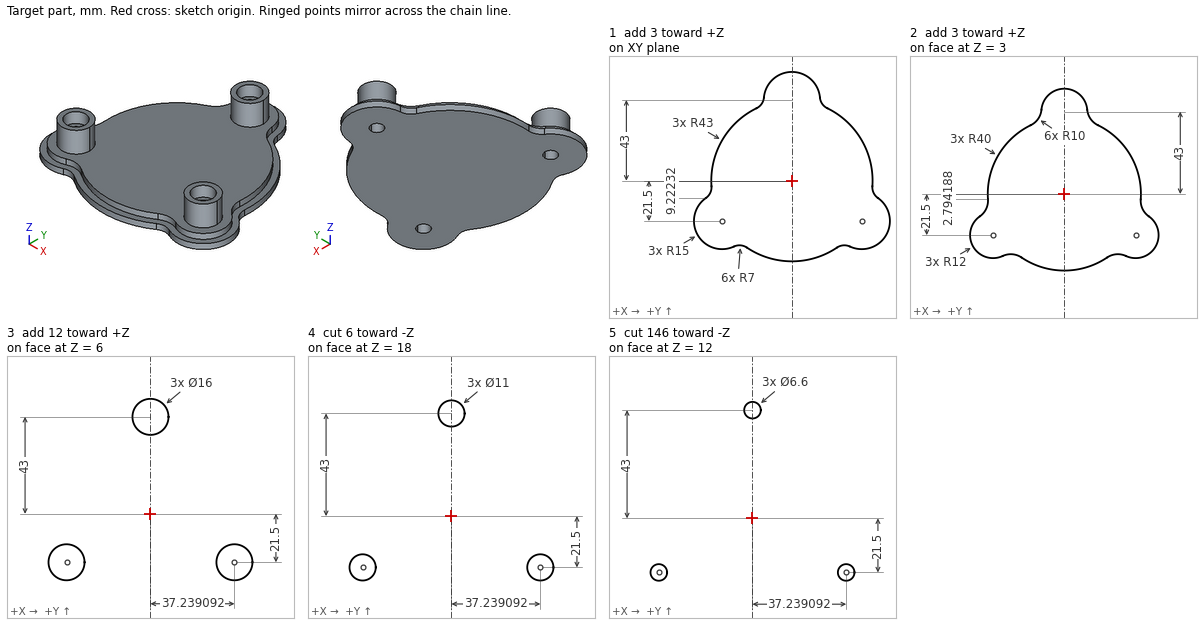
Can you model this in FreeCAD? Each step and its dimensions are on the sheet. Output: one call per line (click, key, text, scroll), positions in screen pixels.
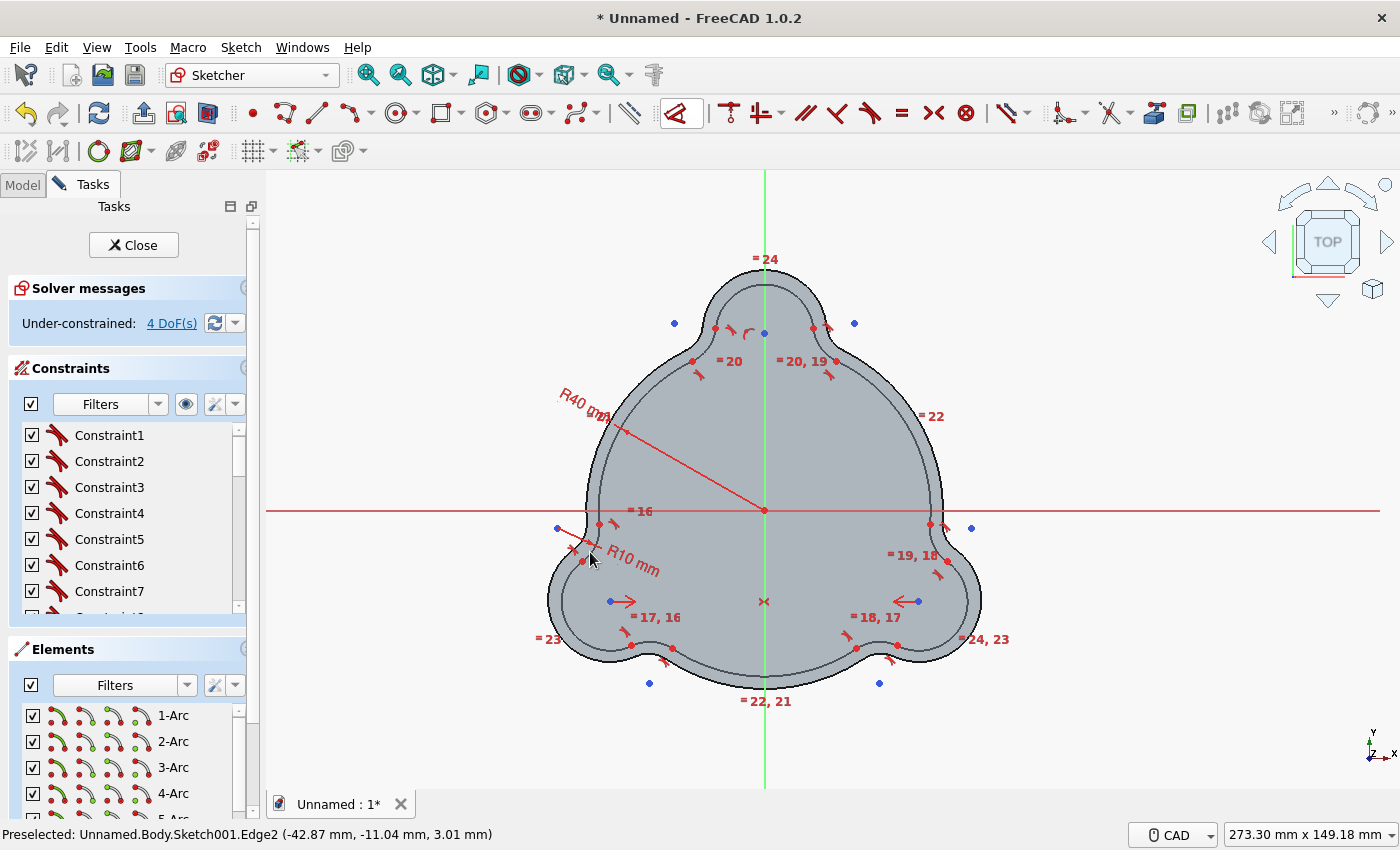
click(562, 599)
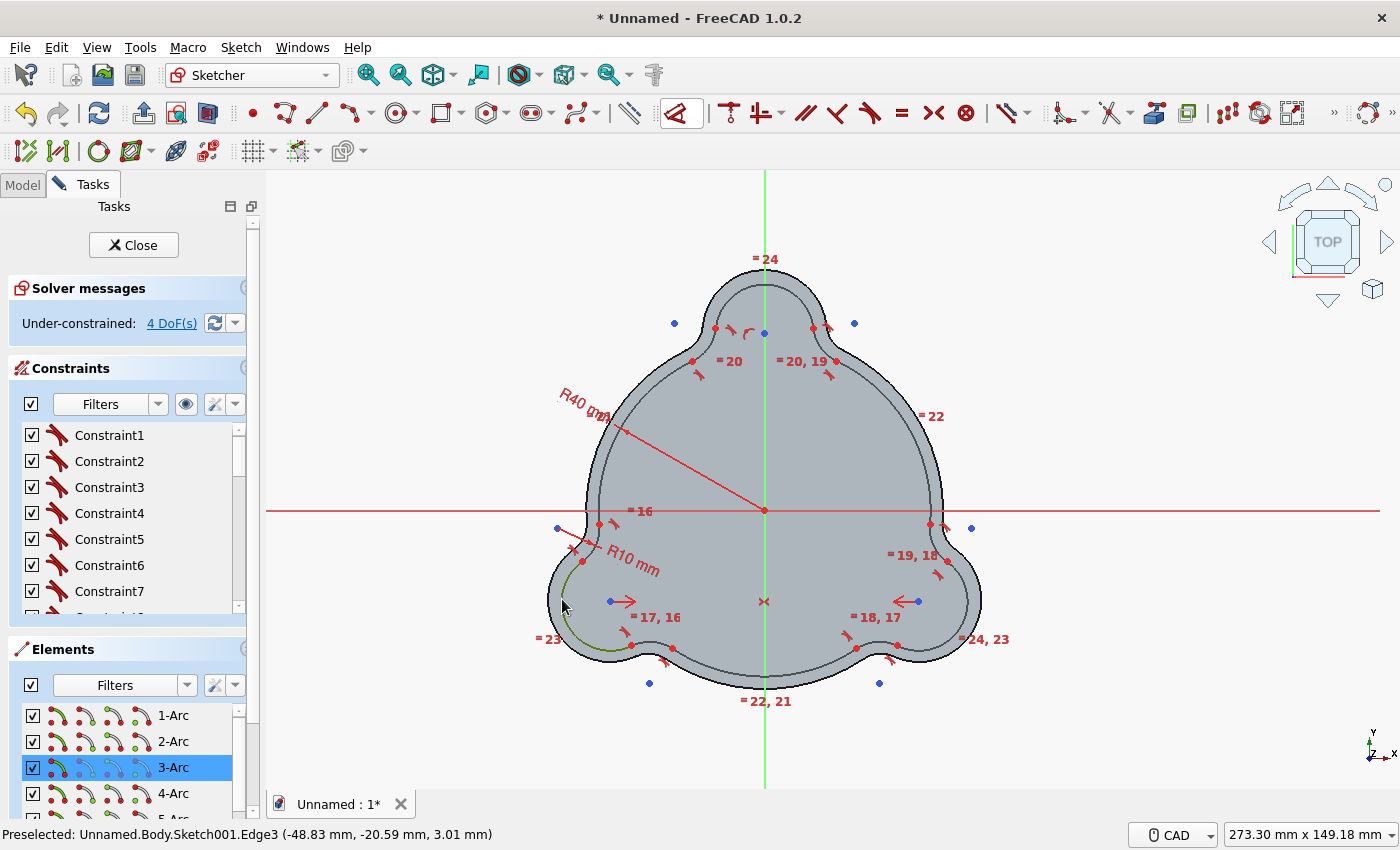
key(k)
key(r)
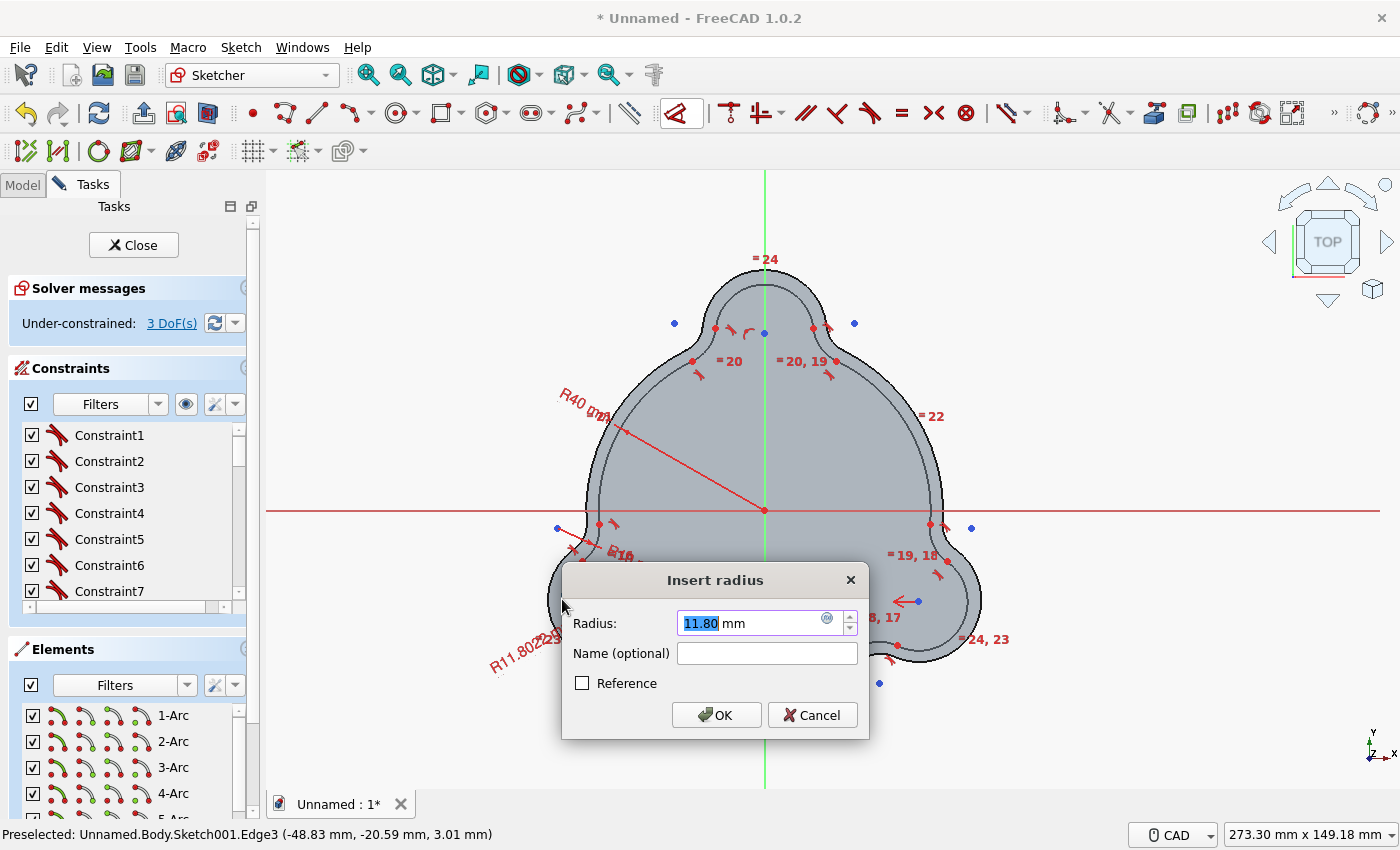
text(12)
key(Return)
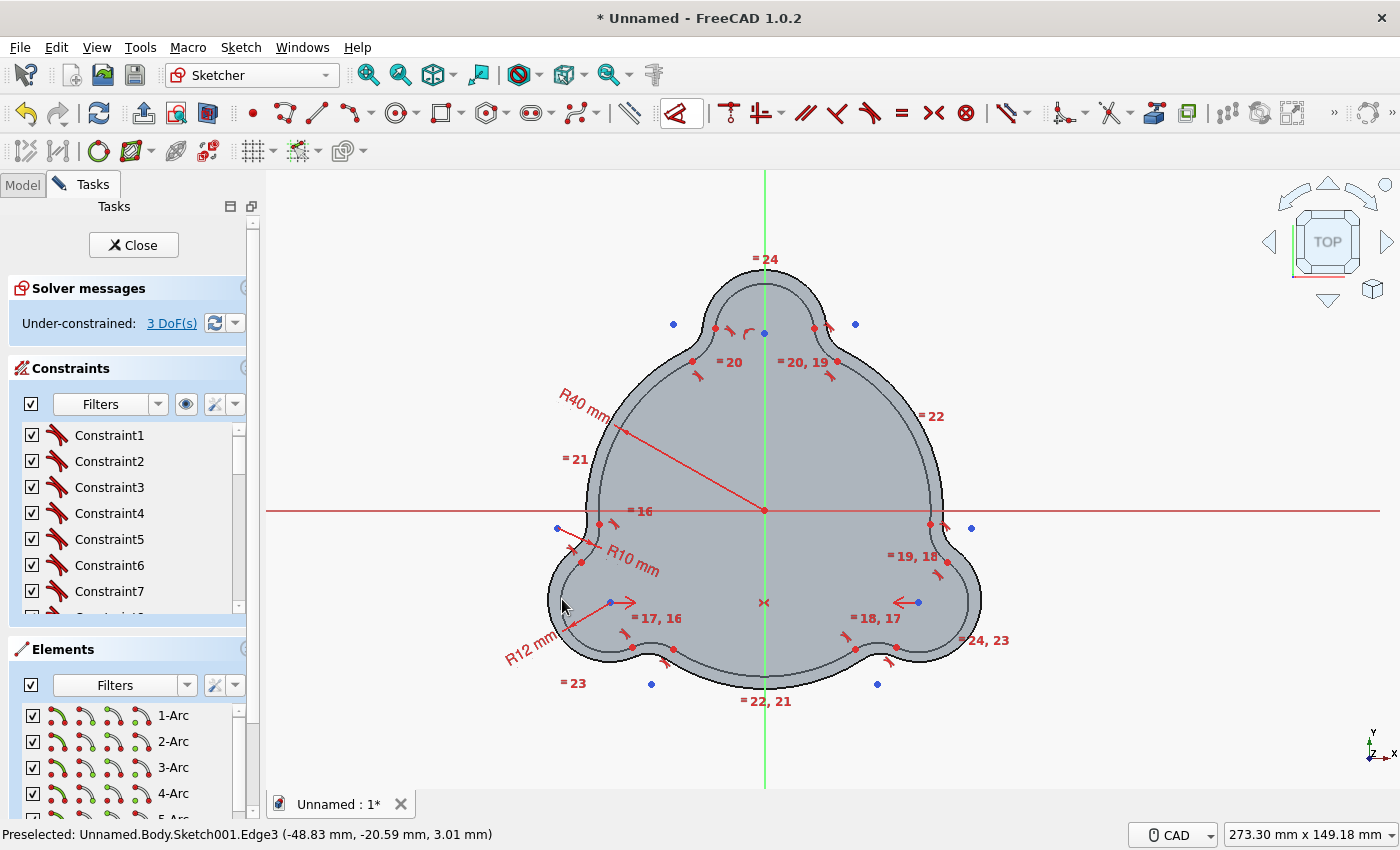
click(765, 334)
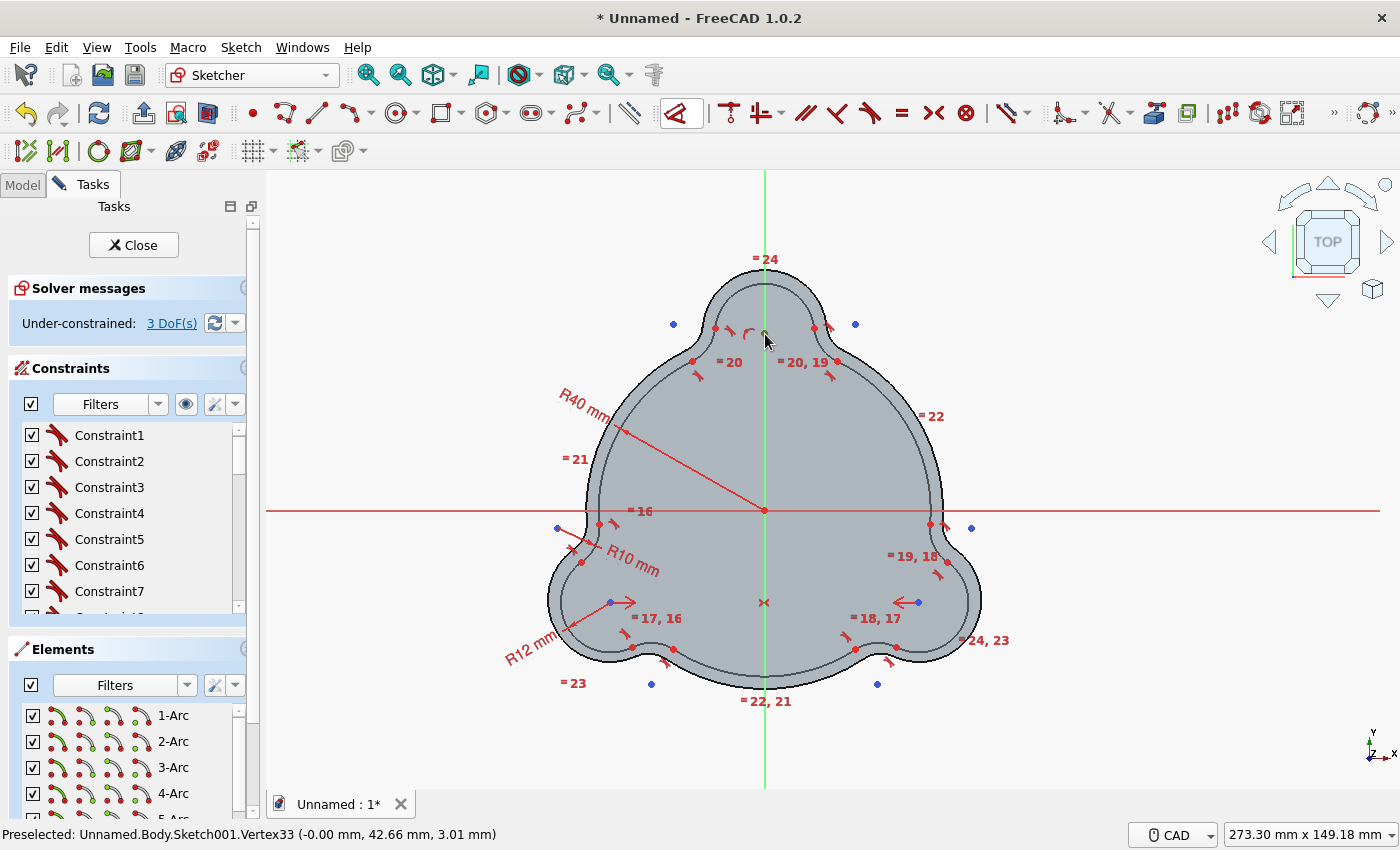
key(i)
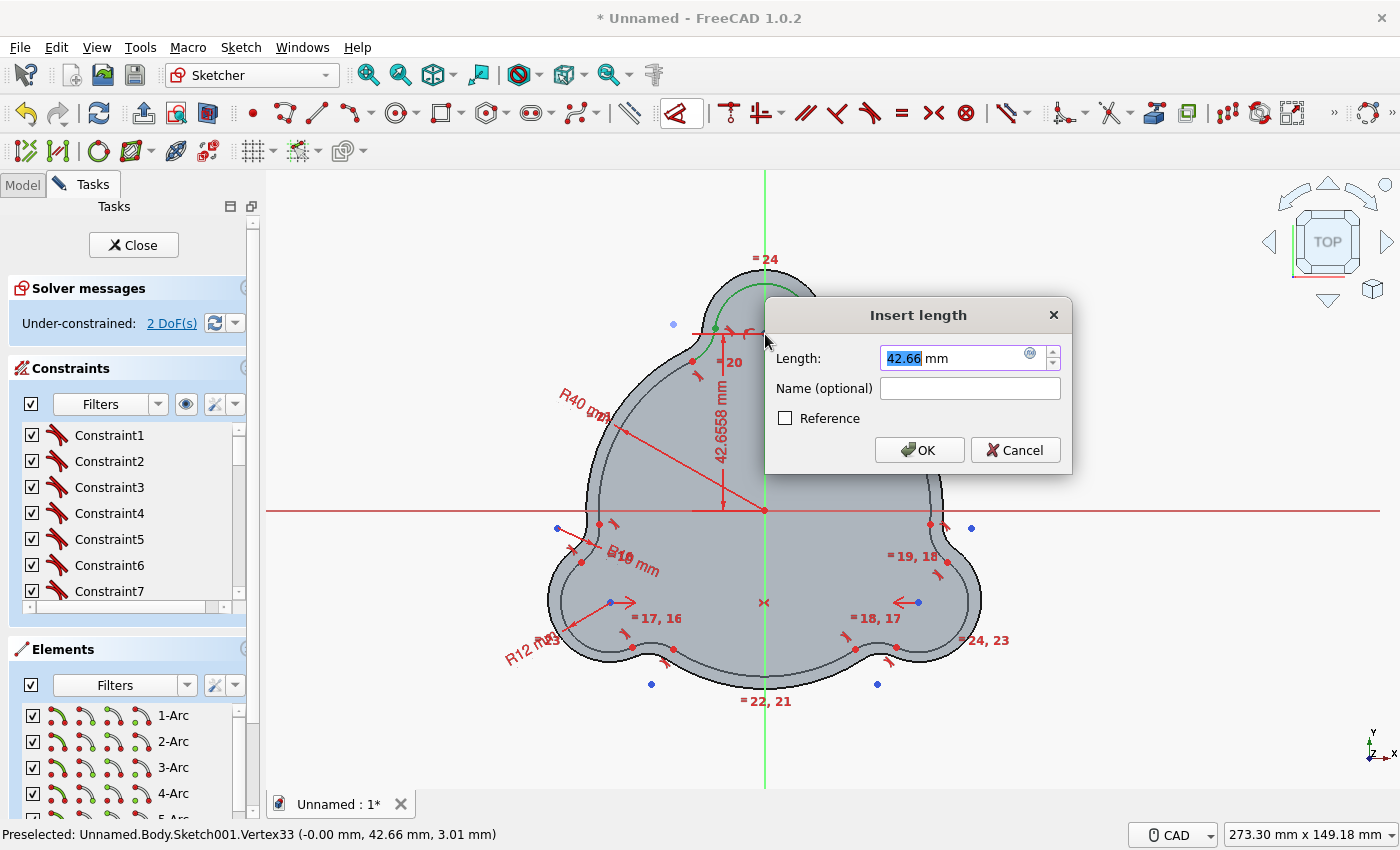
text(43)
key(Return)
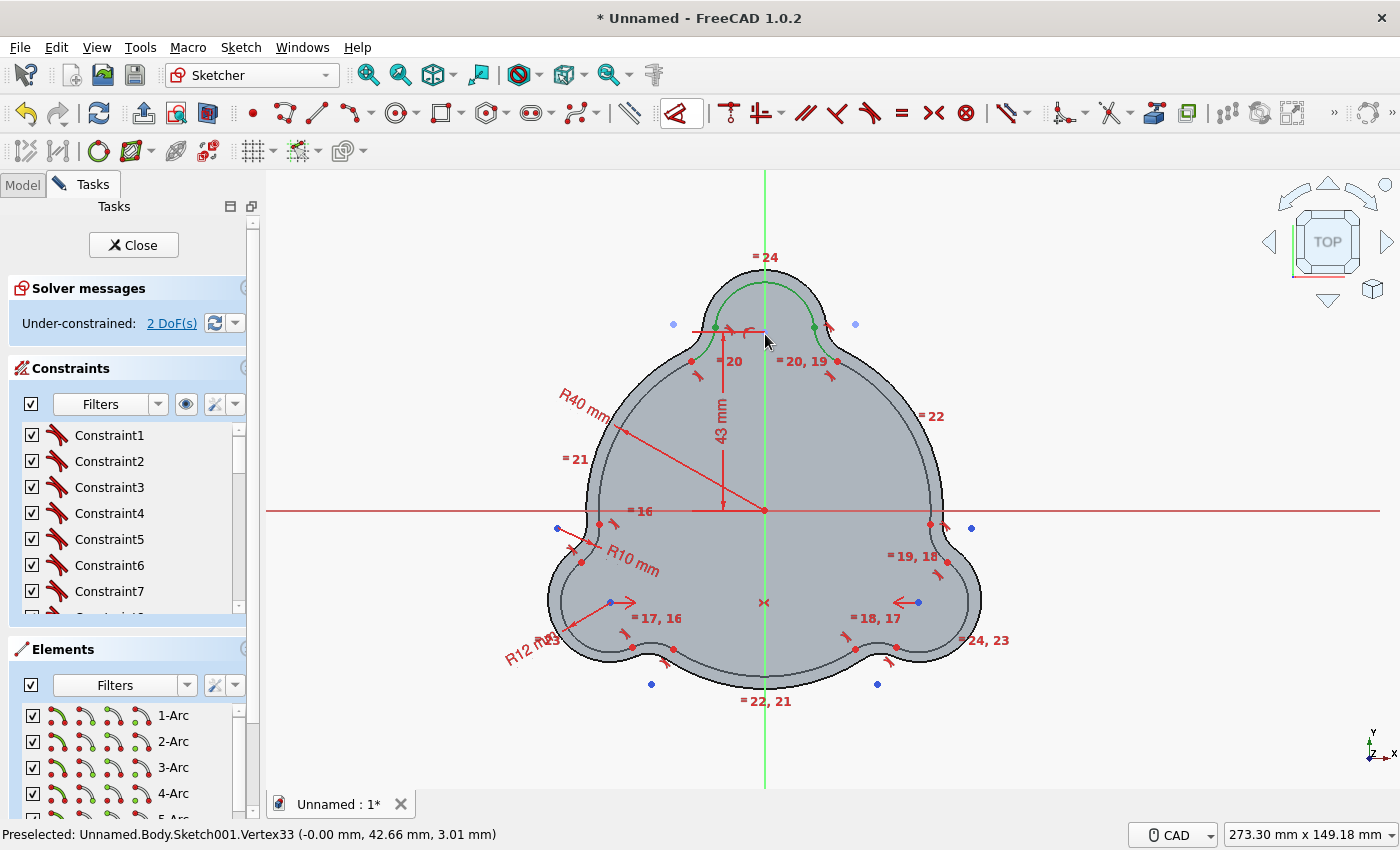
click(611, 603)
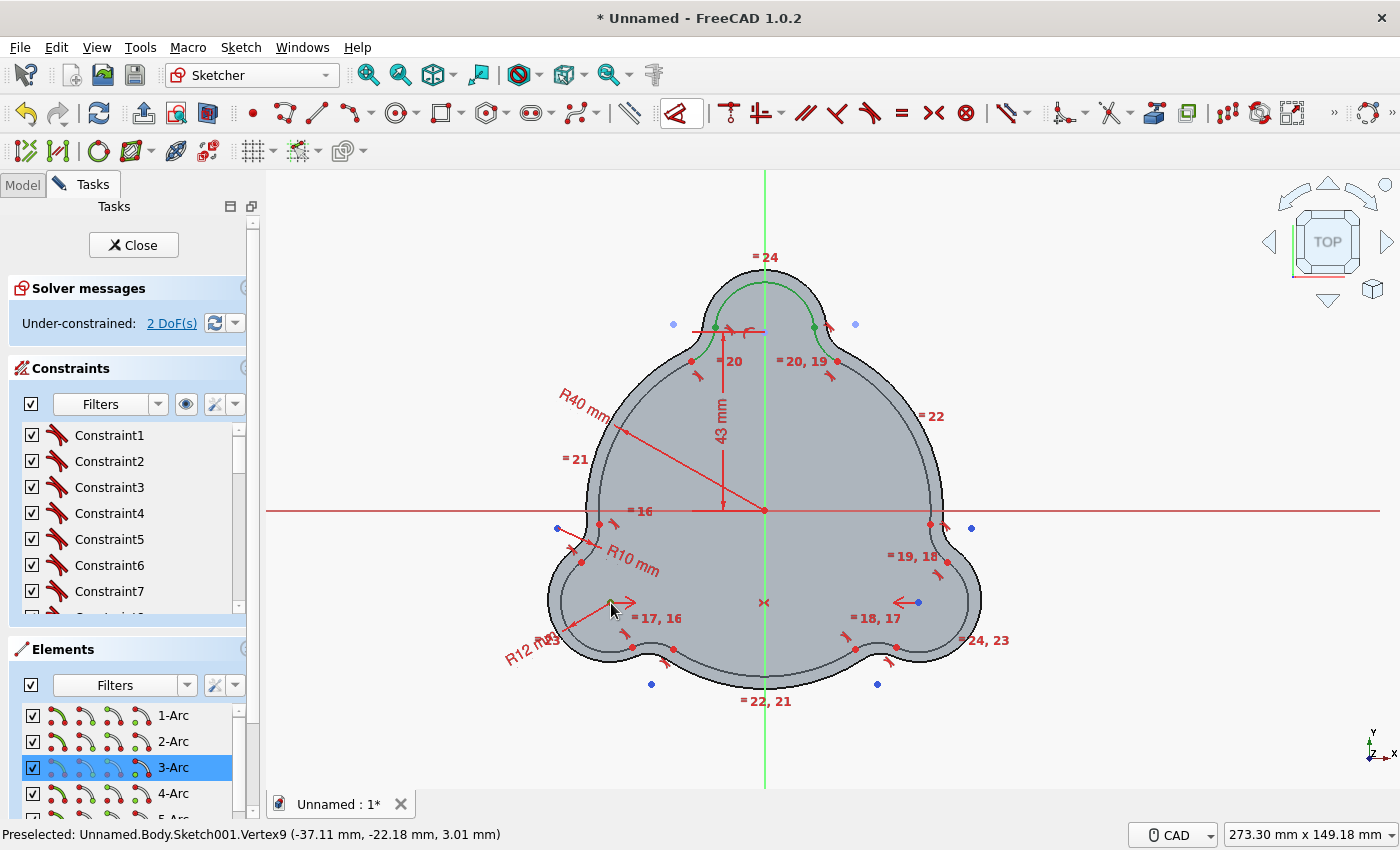
click(698, 114)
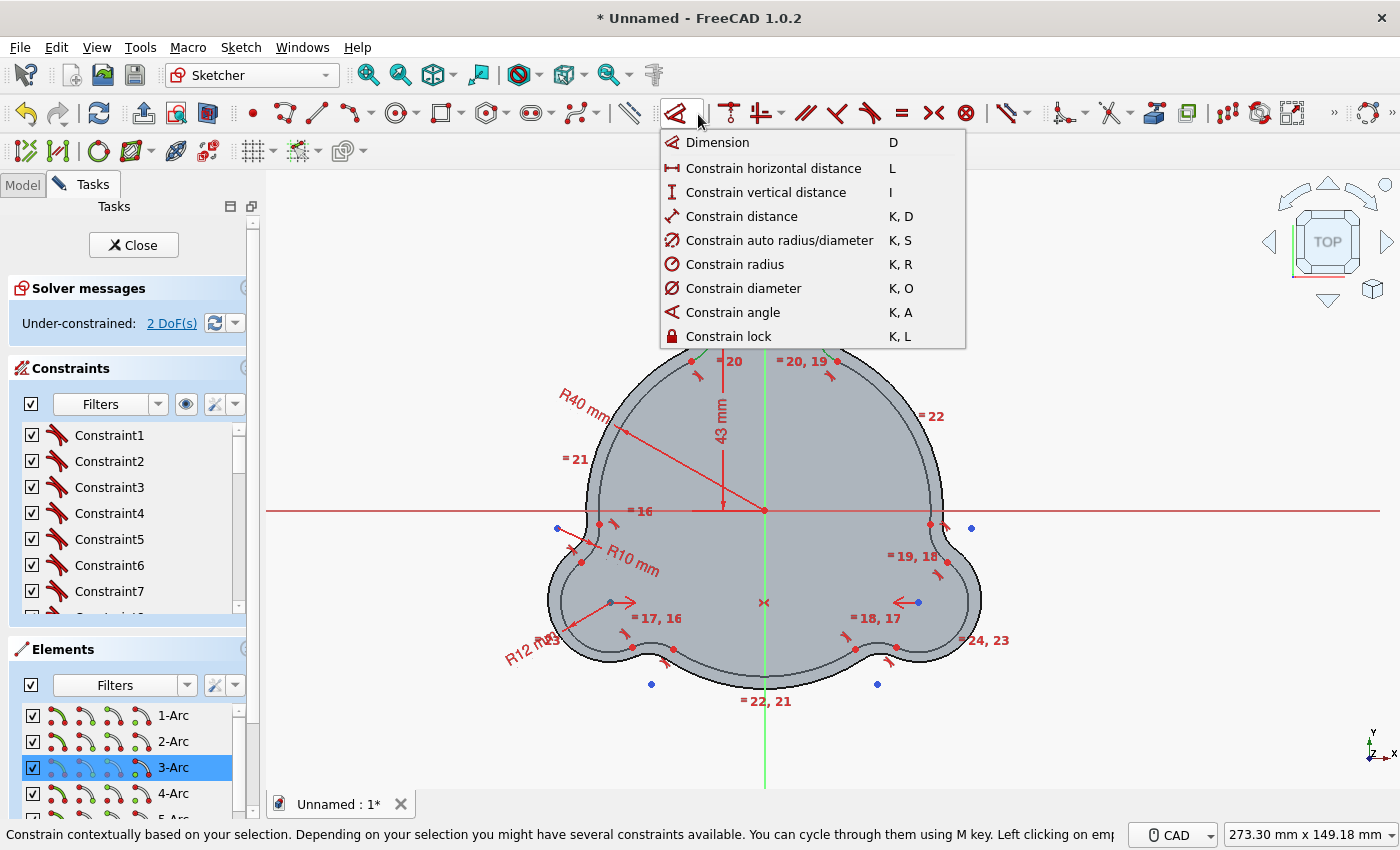
click(813, 192)